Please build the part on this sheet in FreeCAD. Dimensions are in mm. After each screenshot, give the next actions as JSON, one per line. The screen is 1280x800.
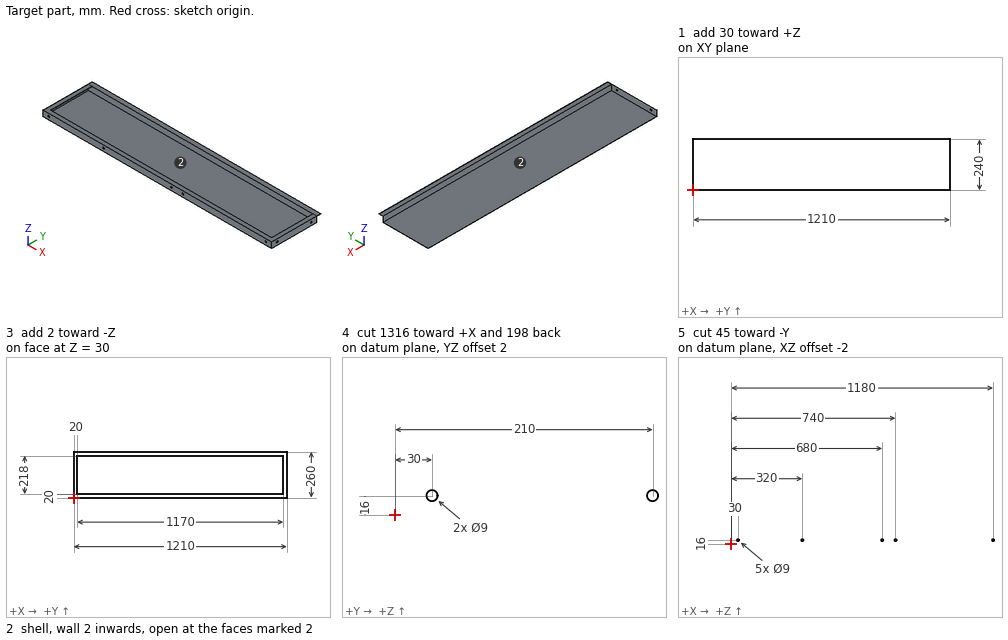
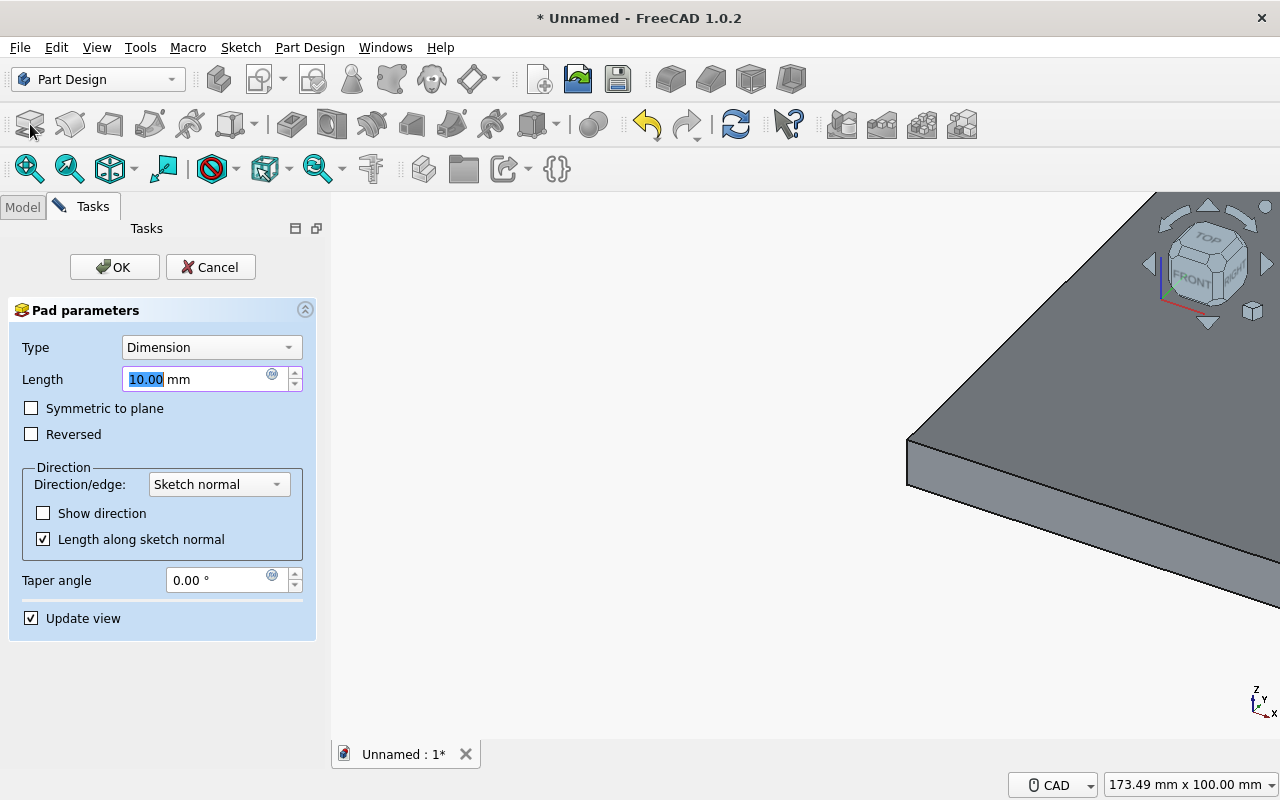
{"action": "type", "text": "30"}
{"action": "key", "text": "Tab"}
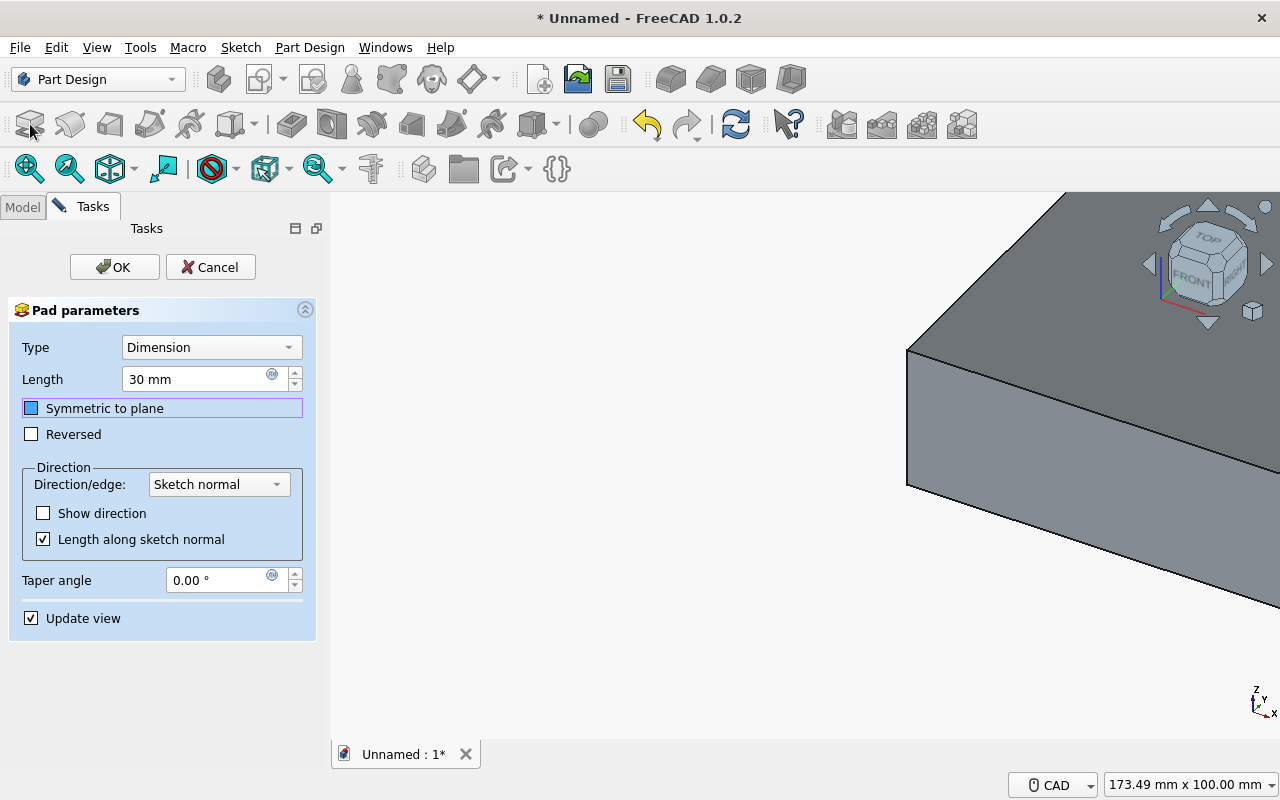
{"action": "left_click", "coordinate": [115, 267]}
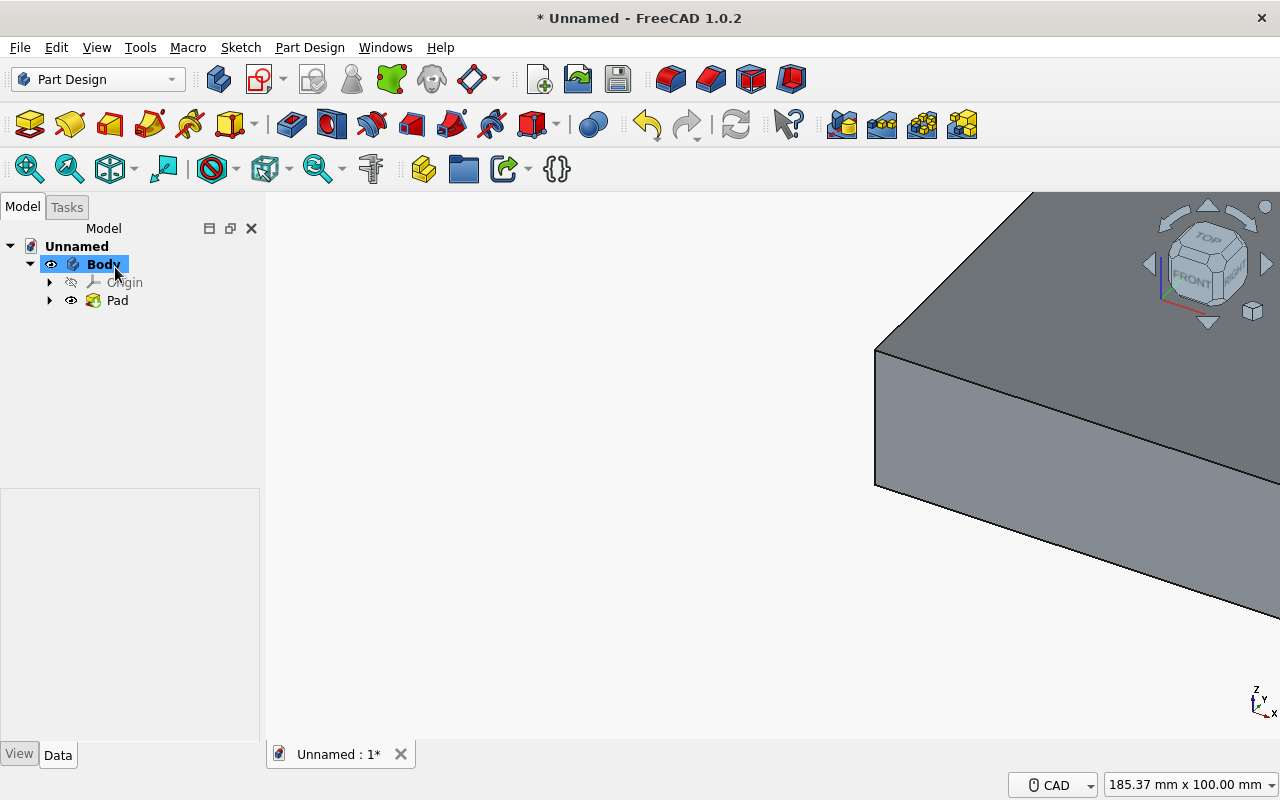
{"action": "left_click", "coordinate": [30, 170]}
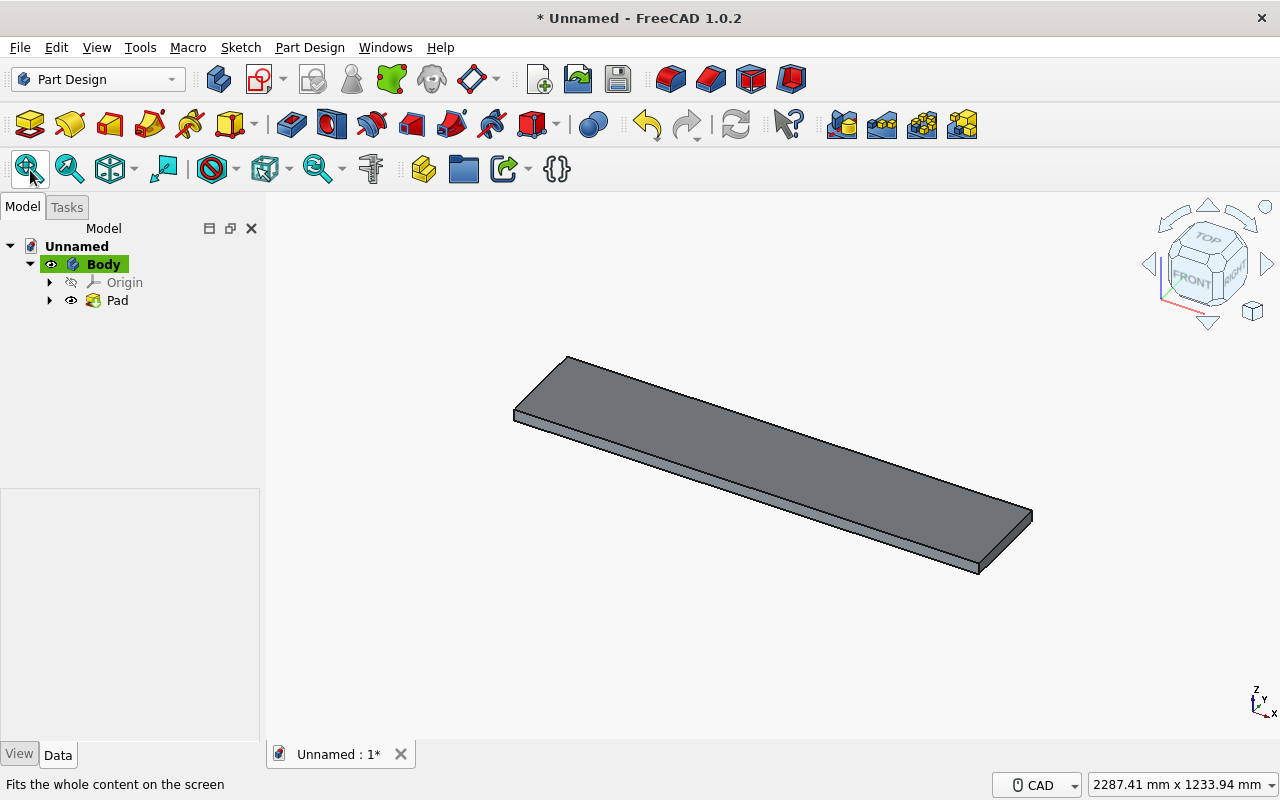
{"action": "left_click", "coordinate": [906, 503]}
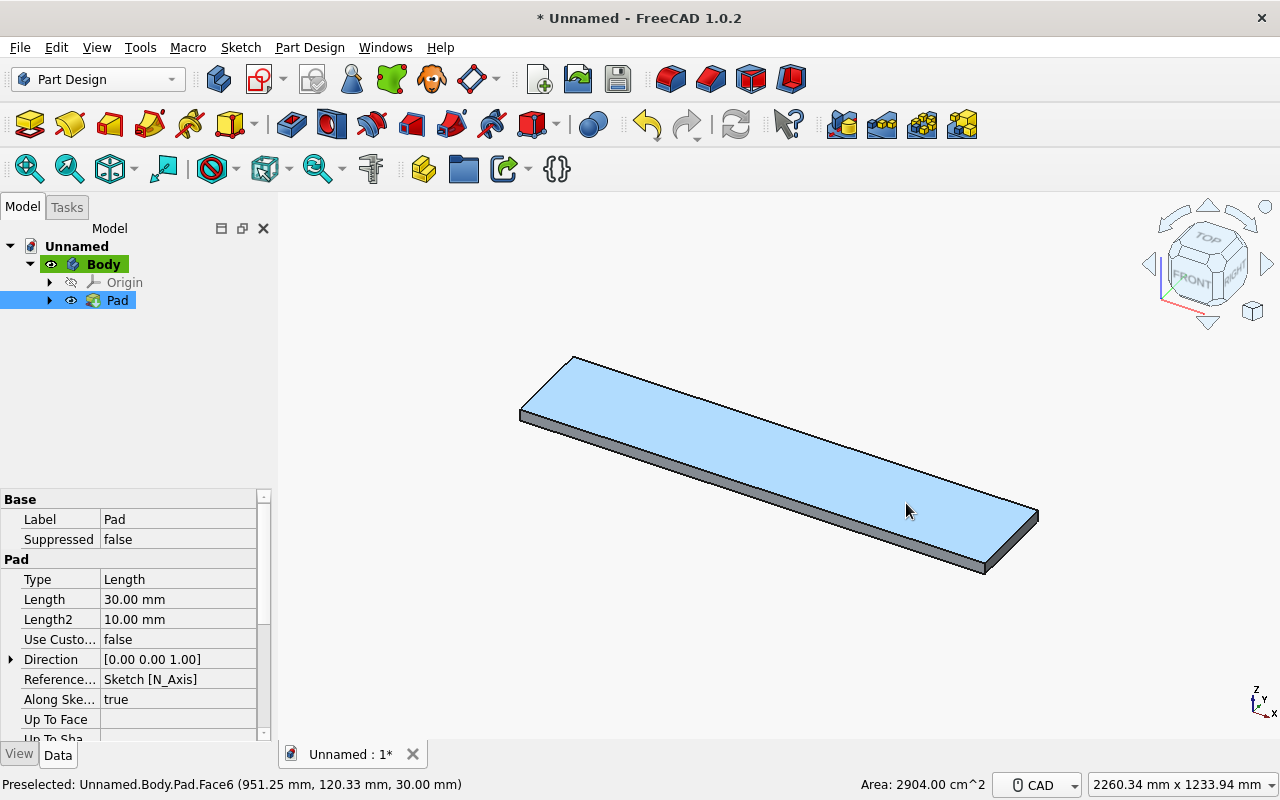
{"action": "left_click", "coordinate": [792, 80]}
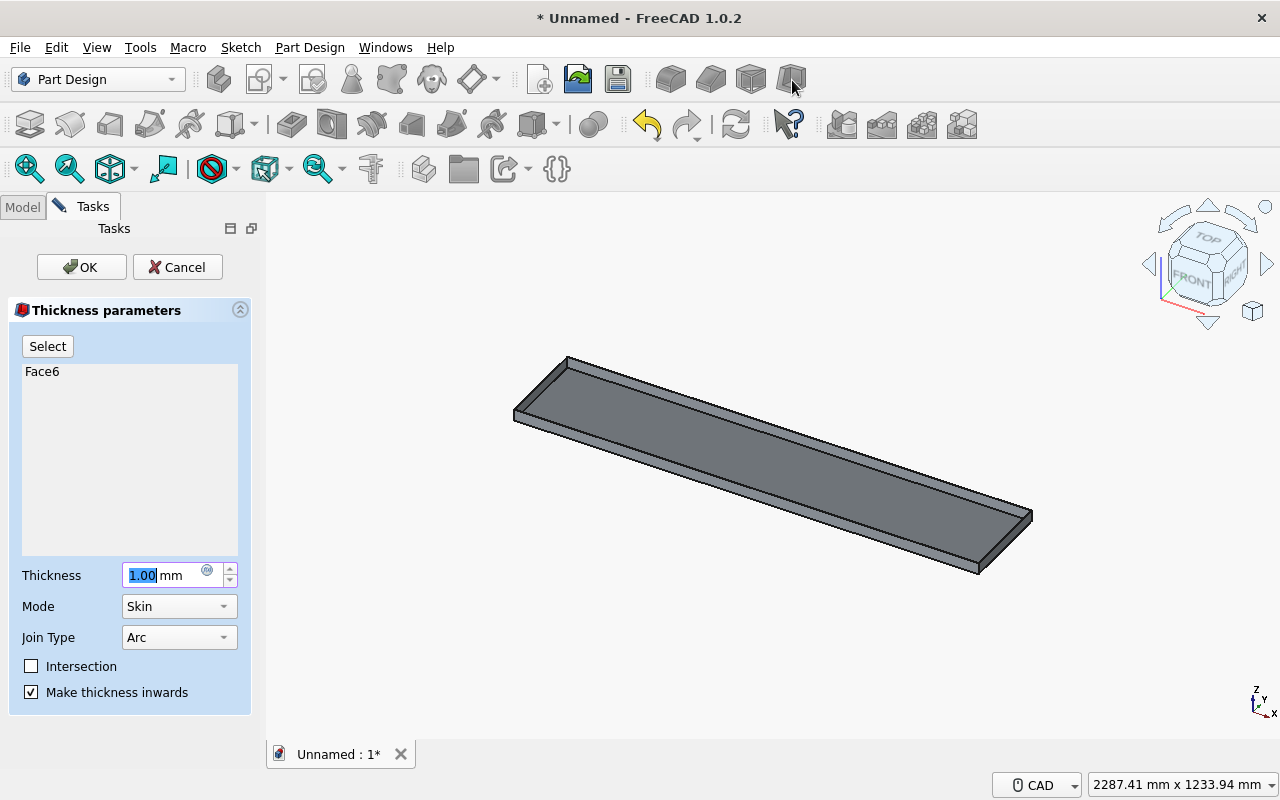
{"action": "type", "text": "2"}
{"action": "key", "text": "Tab"}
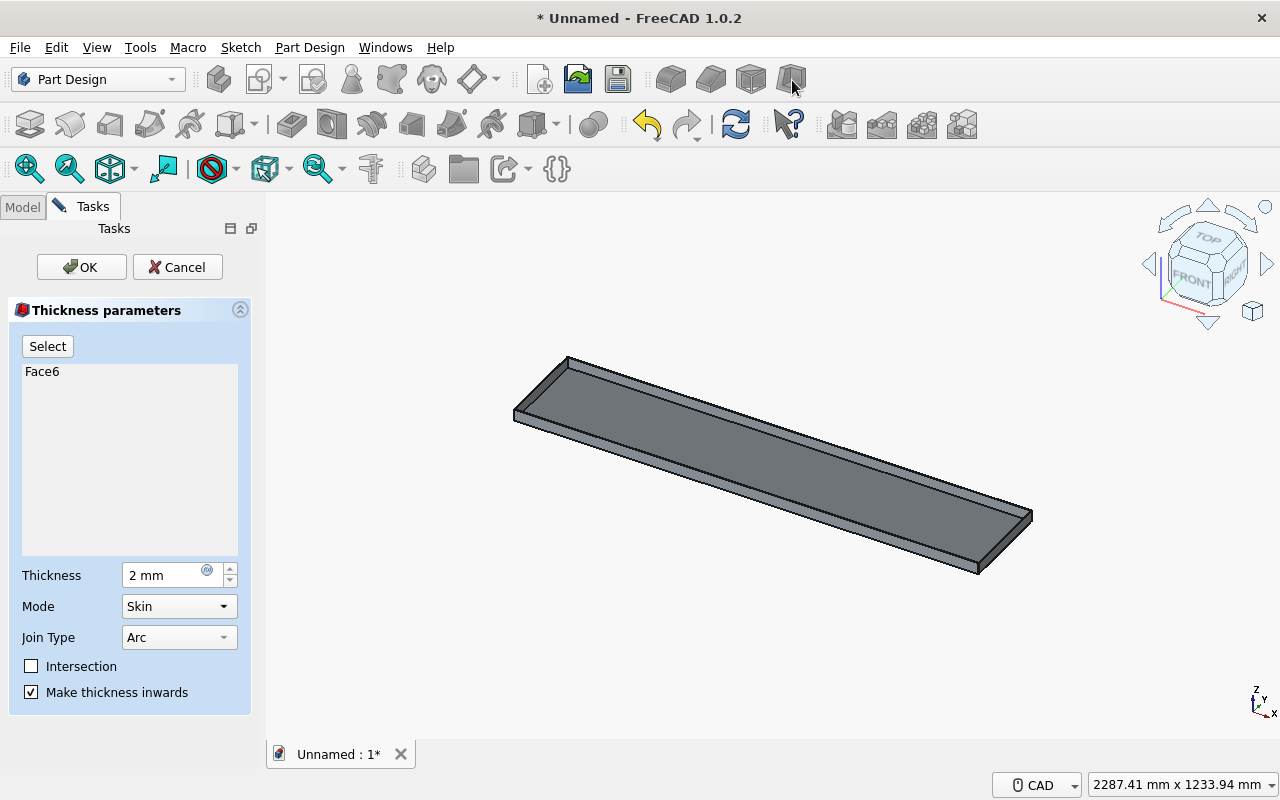
{"action": "left_click", "coordinate": [180, 638]}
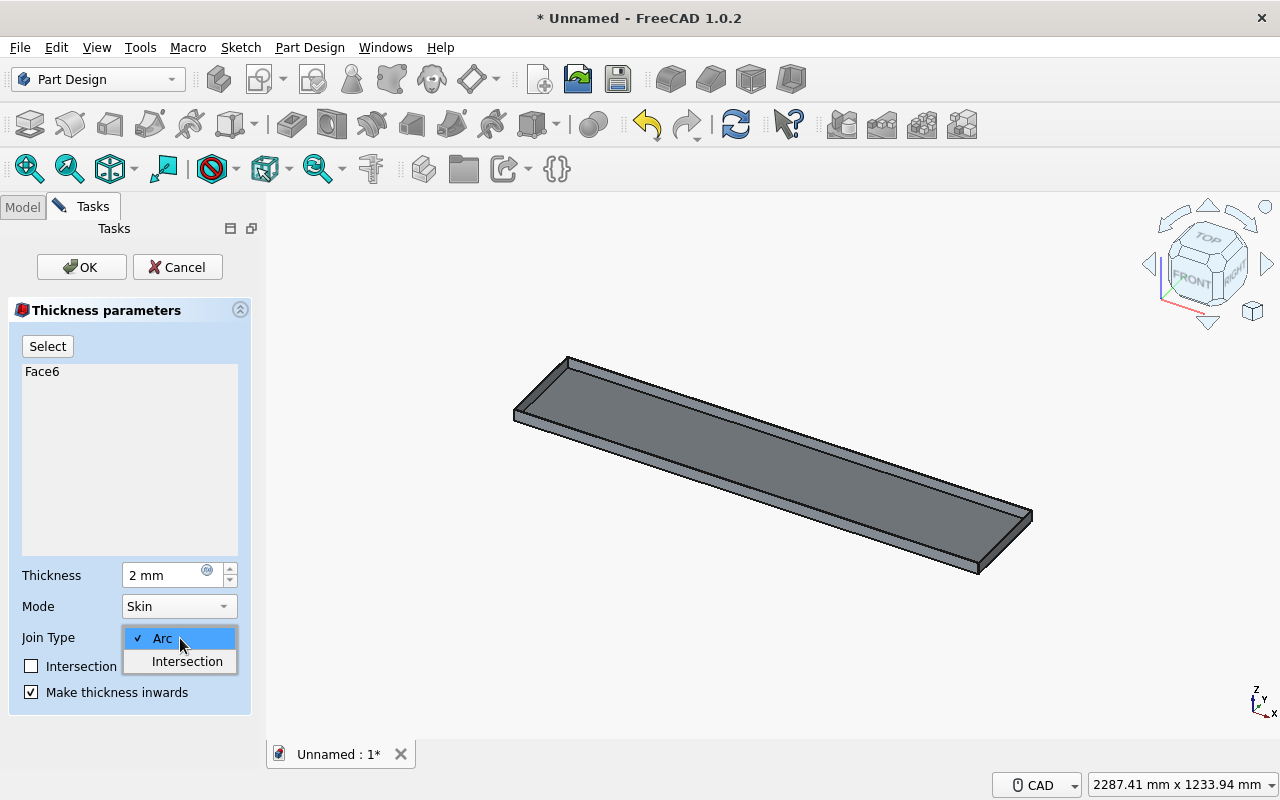
{"action": "left_click", "coordinate": [179, 662]}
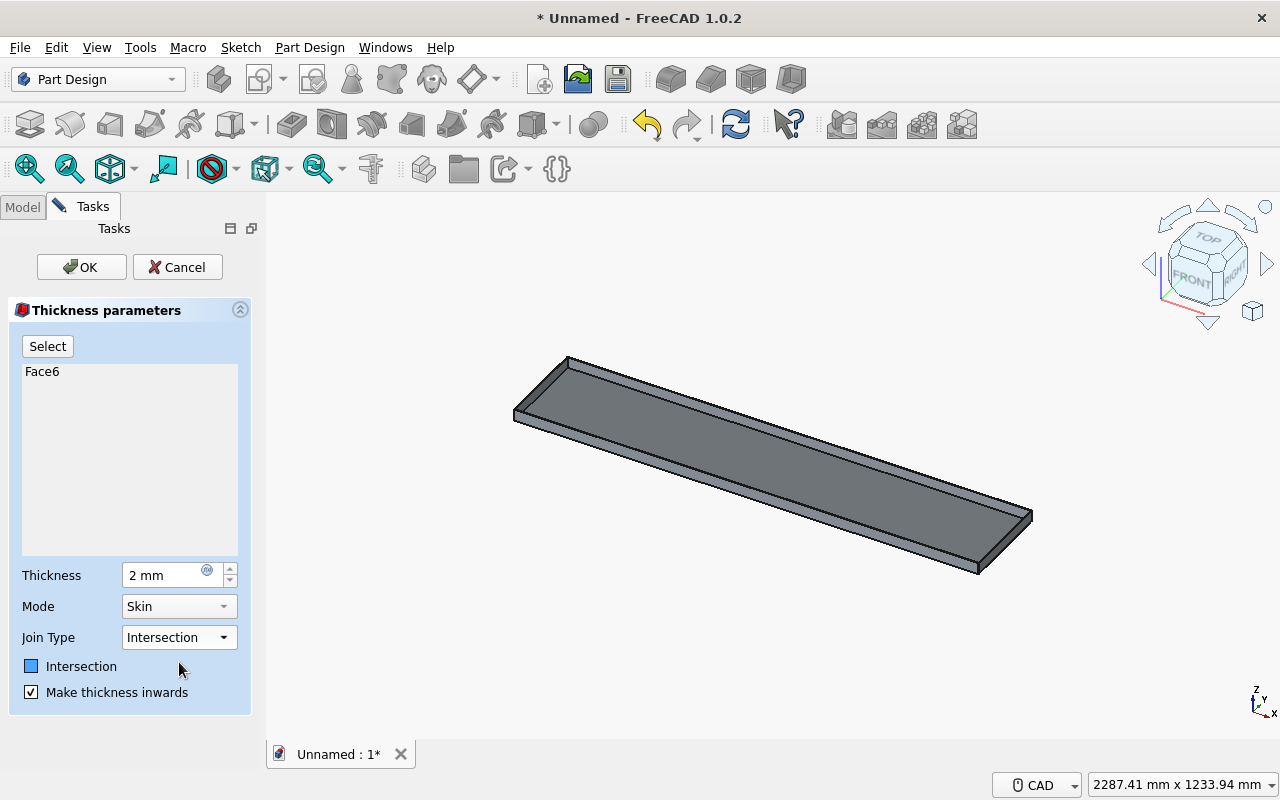
{"action": "left_click", "coordinate": [82, 267]}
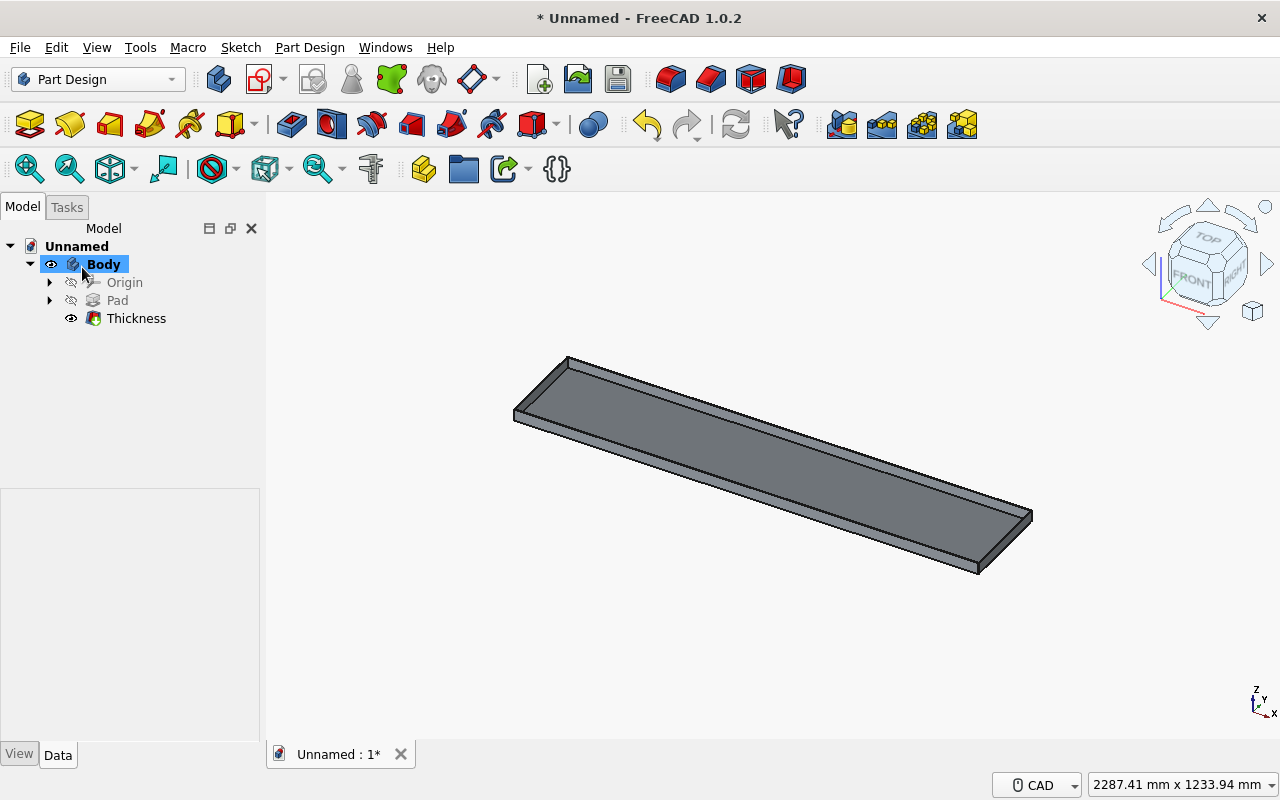
{"action": "scroll", "coordinate": [1014, 527], "scroll_direction": "up", "scroll_amount": 15}